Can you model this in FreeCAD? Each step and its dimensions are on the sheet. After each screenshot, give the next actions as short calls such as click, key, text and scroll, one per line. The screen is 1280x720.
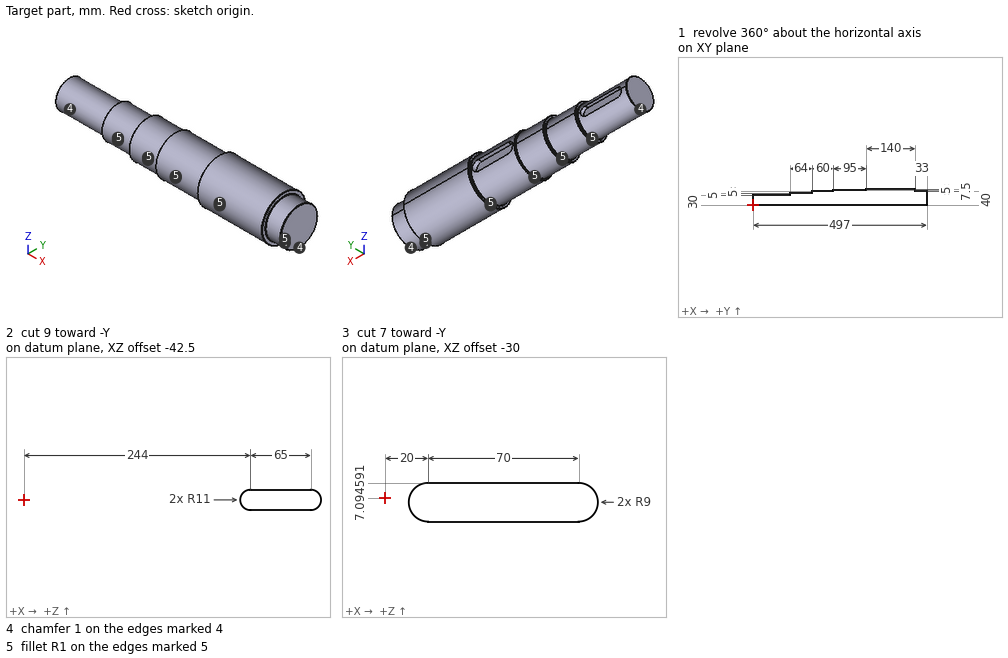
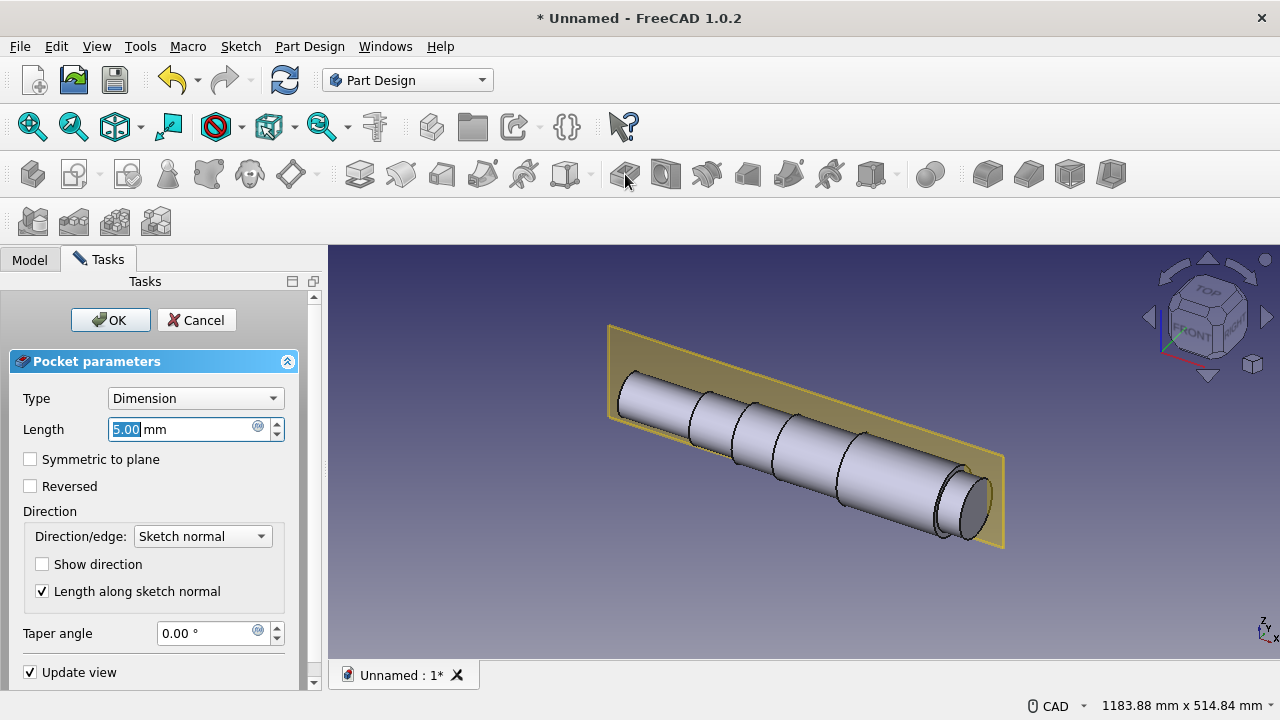
text(7)
key(Tab)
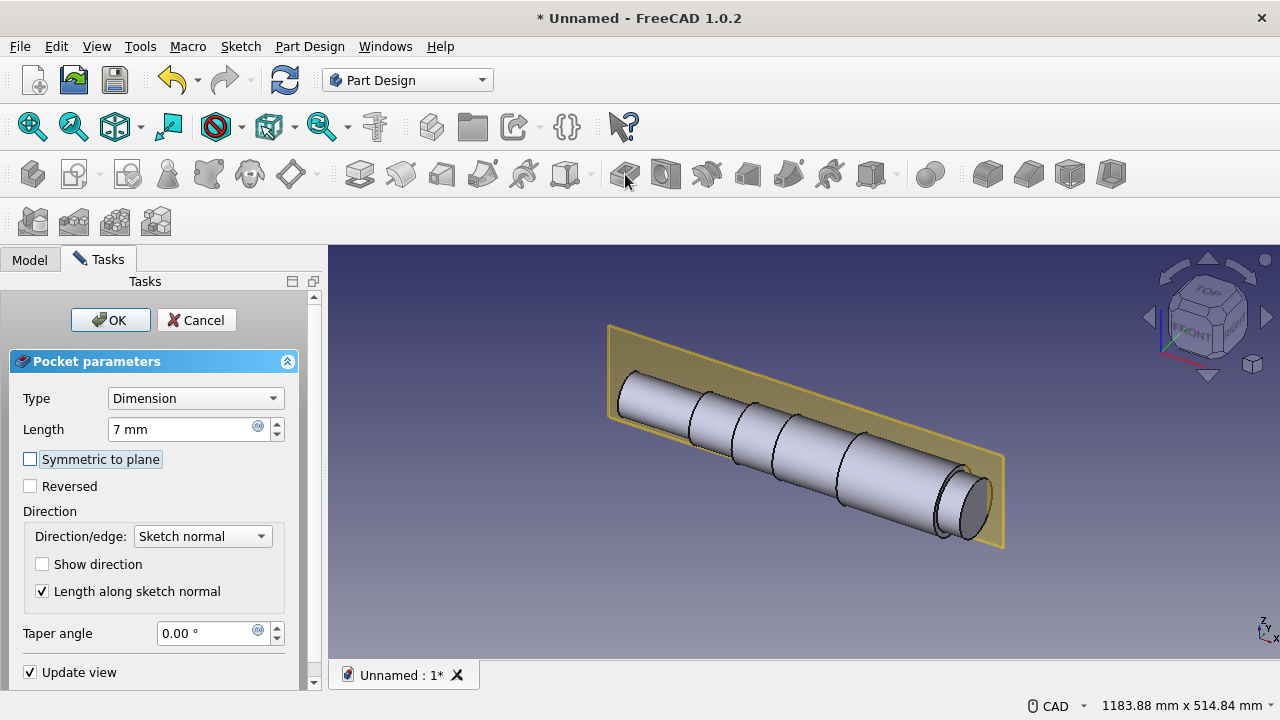
click(31, 486)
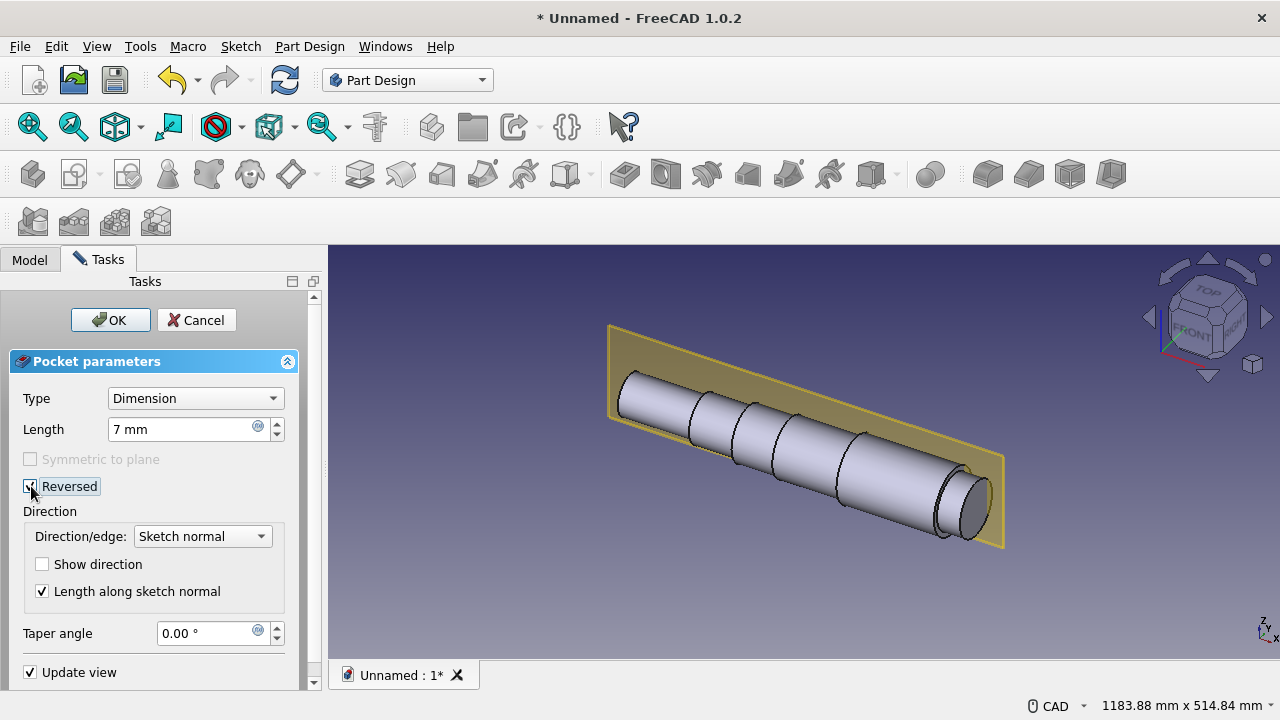
click(111, 320)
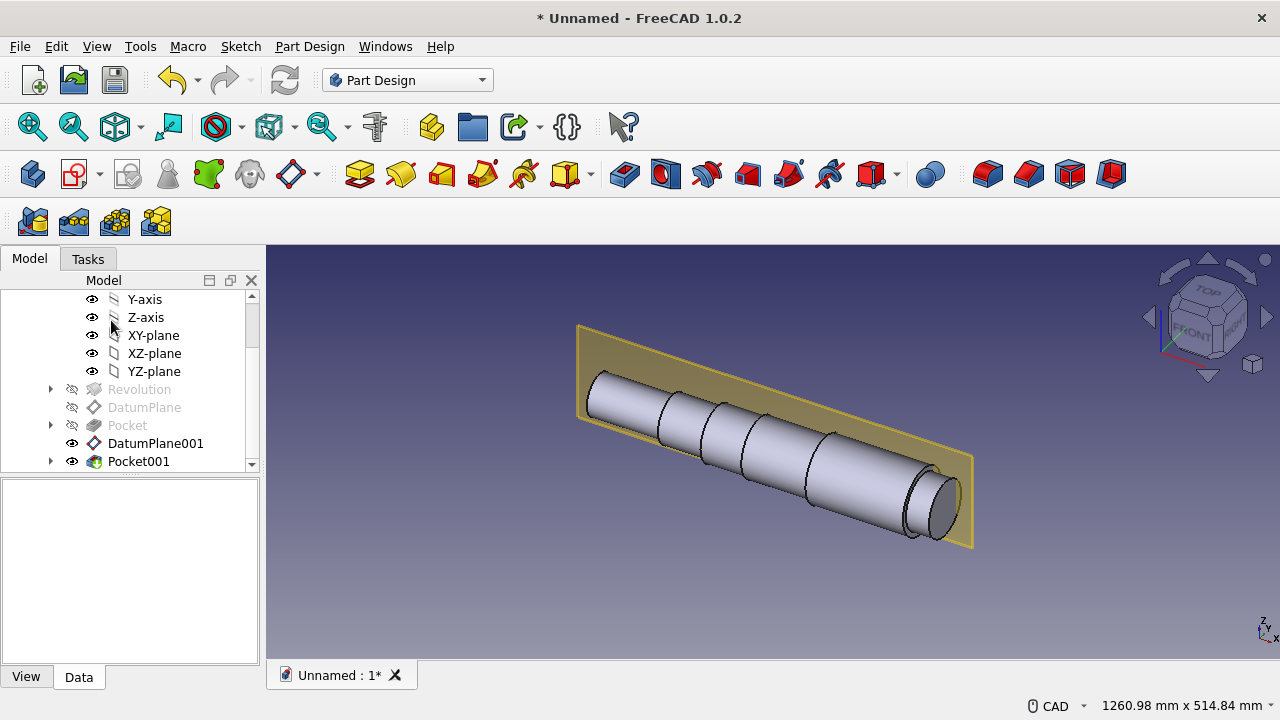
click(117, 443)
key(space)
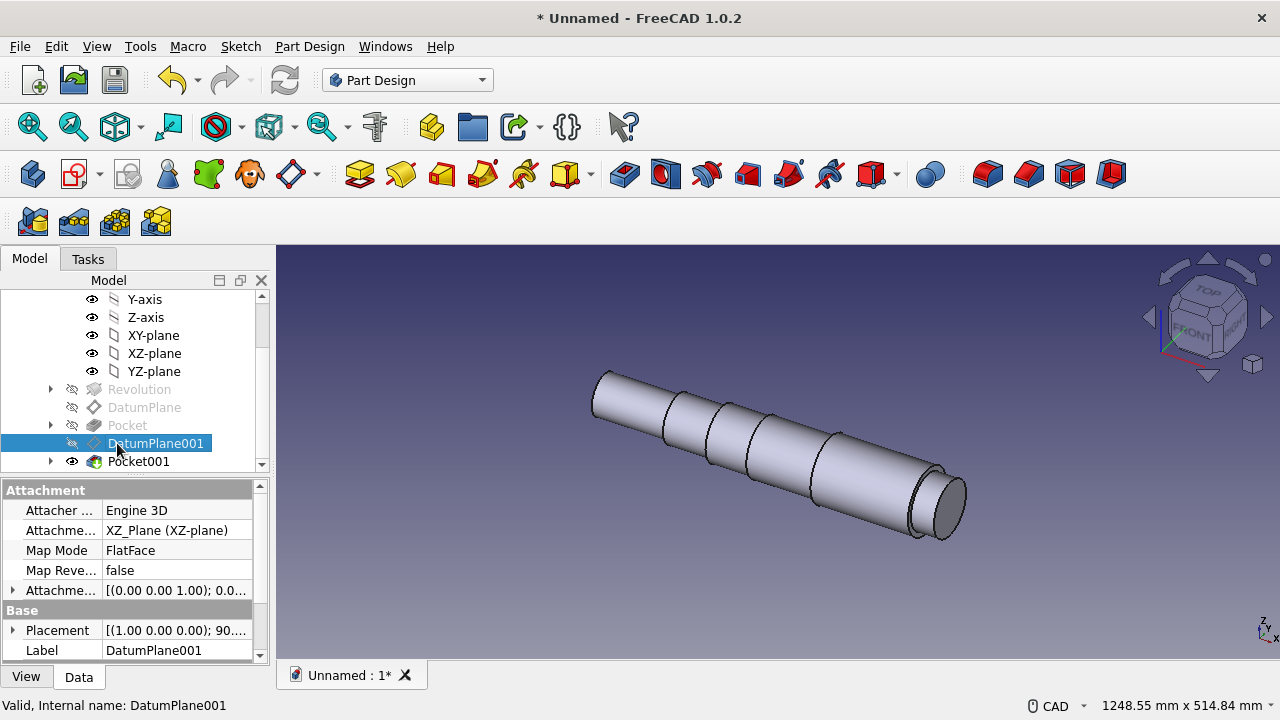
click(934, 524)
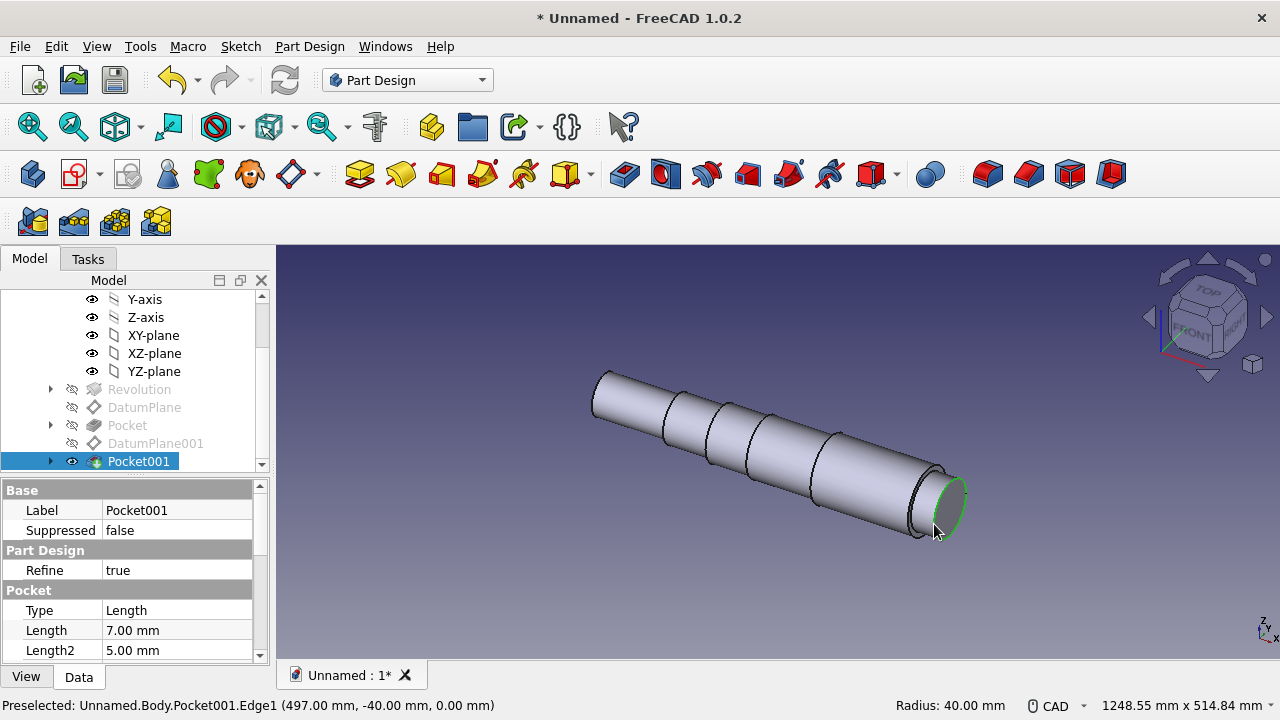
click(908, 519, ctrl)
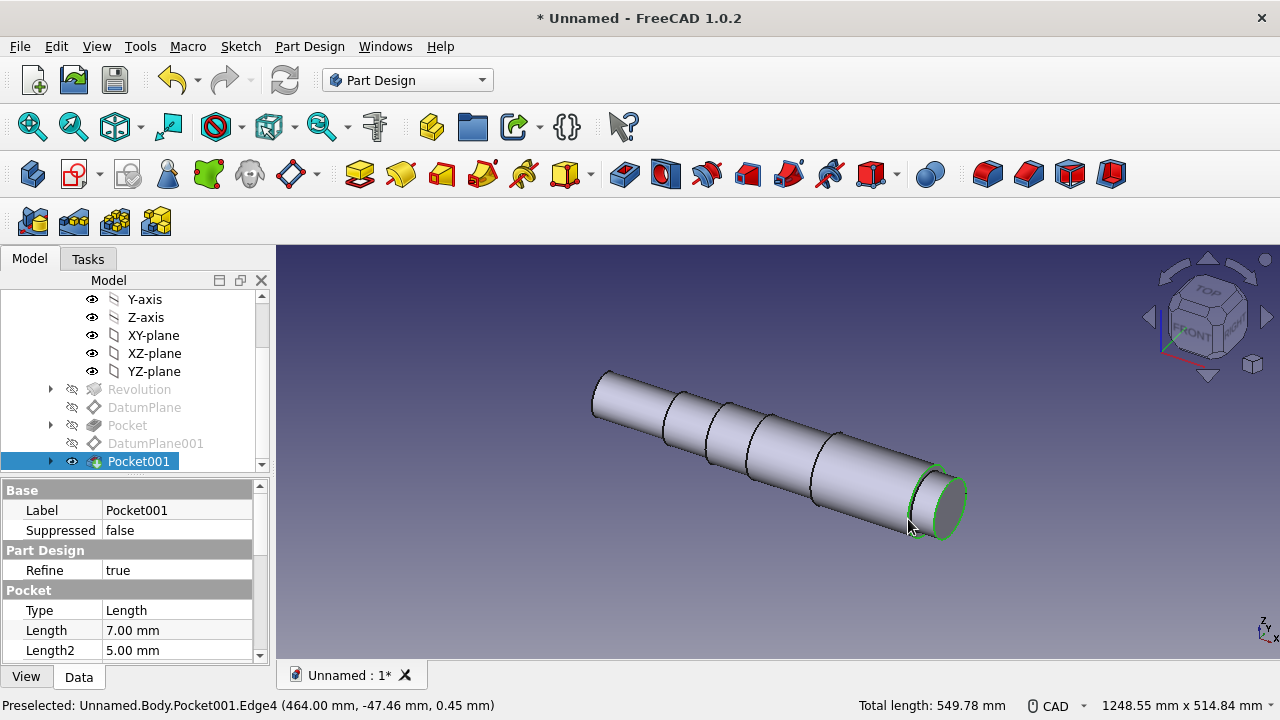
click(824, 444, ctrl)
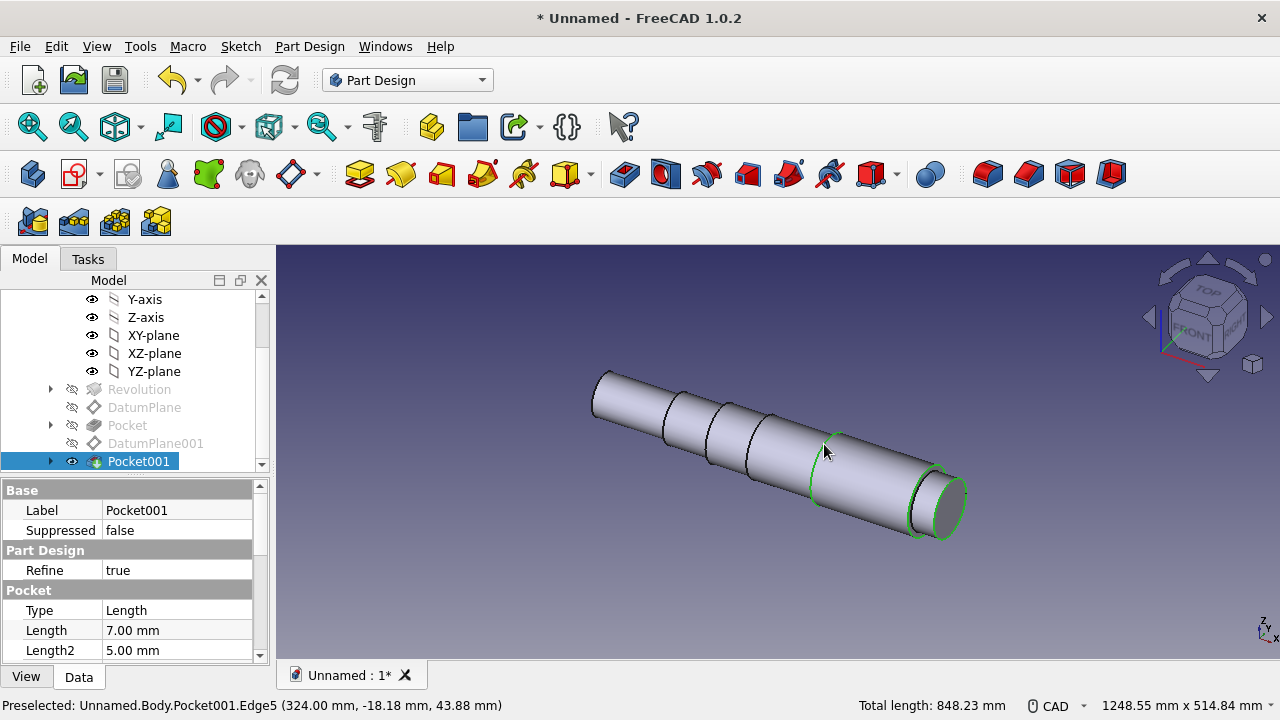
click(746, 463, ctrl)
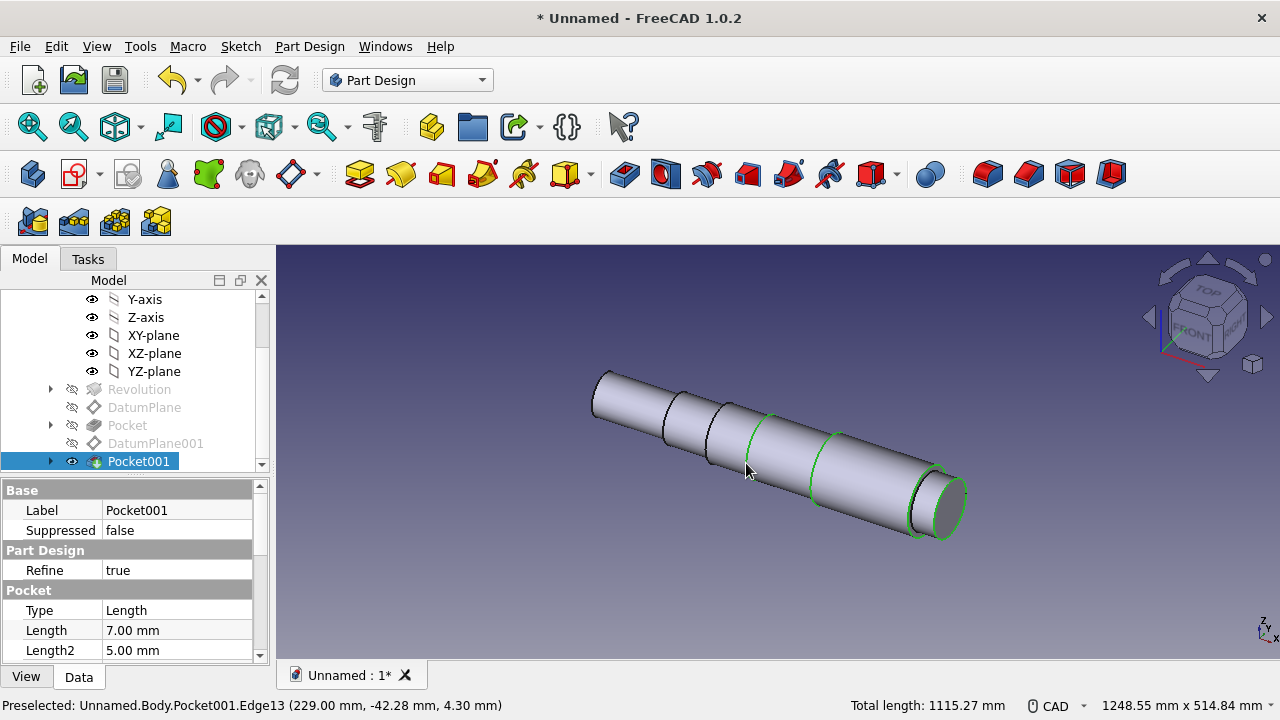
click(705, 448, ctrl)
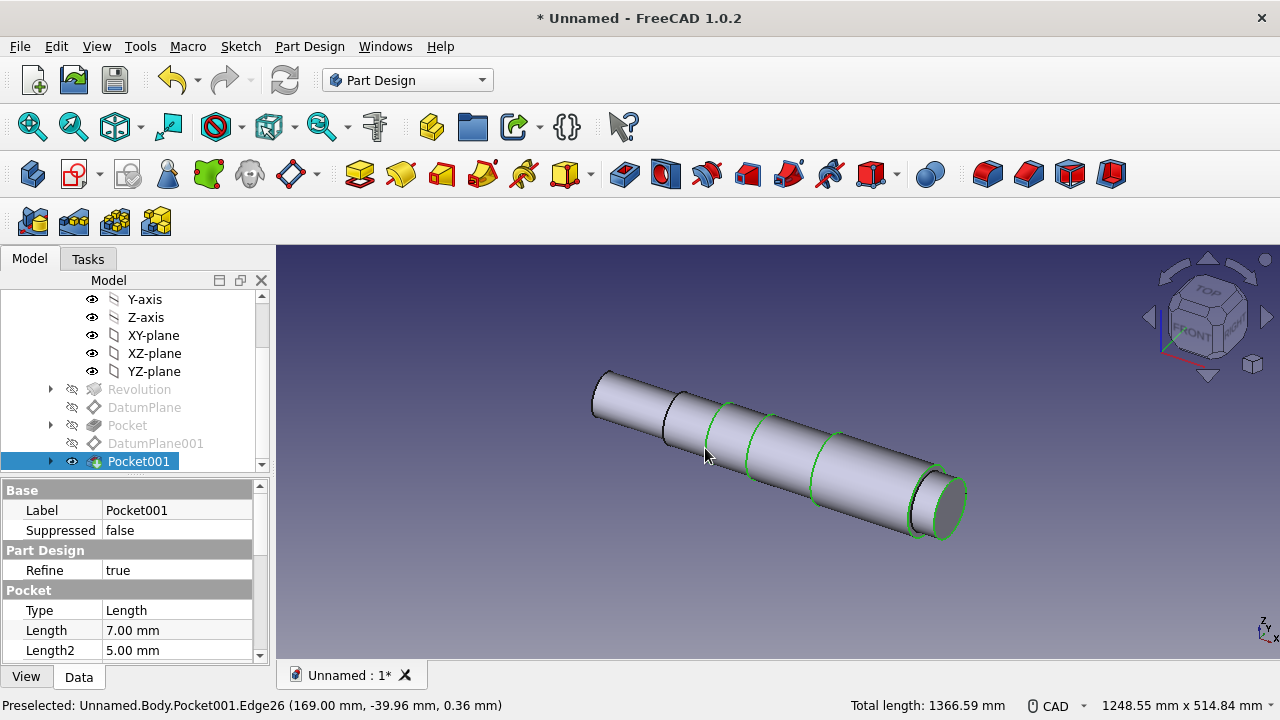
click(681, 391, ctrl)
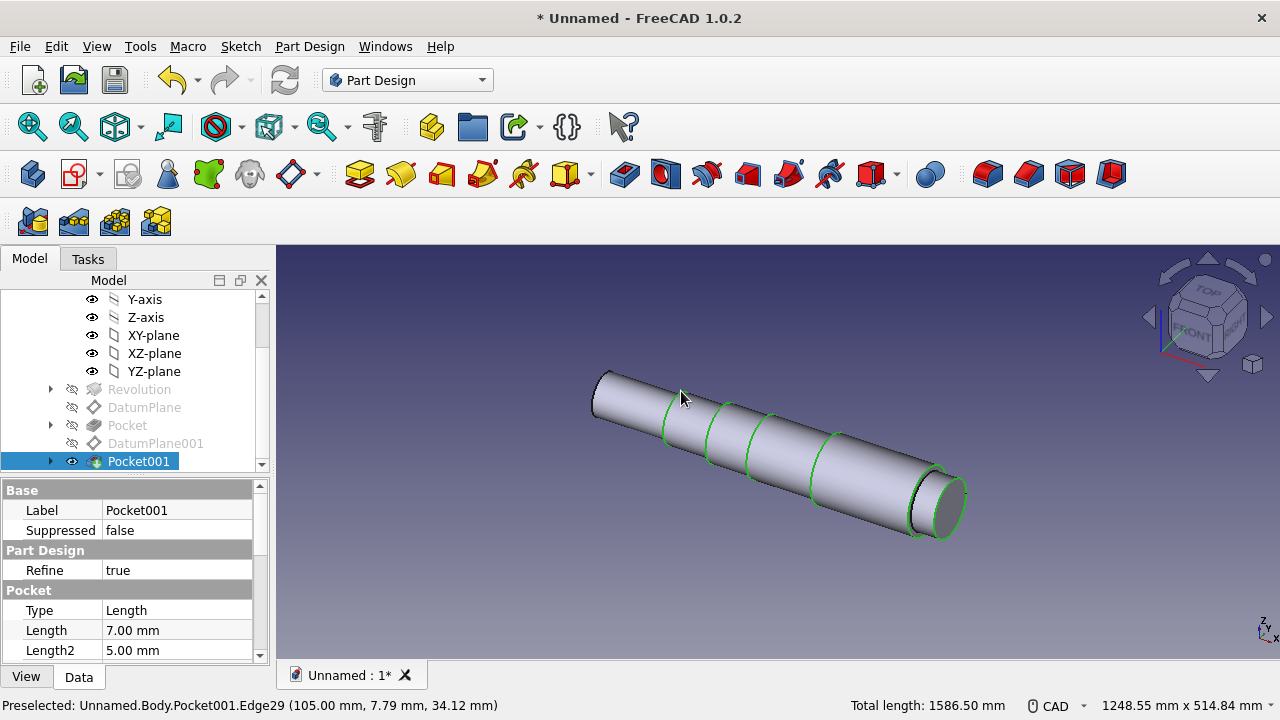
click(594, 415, ctrl)